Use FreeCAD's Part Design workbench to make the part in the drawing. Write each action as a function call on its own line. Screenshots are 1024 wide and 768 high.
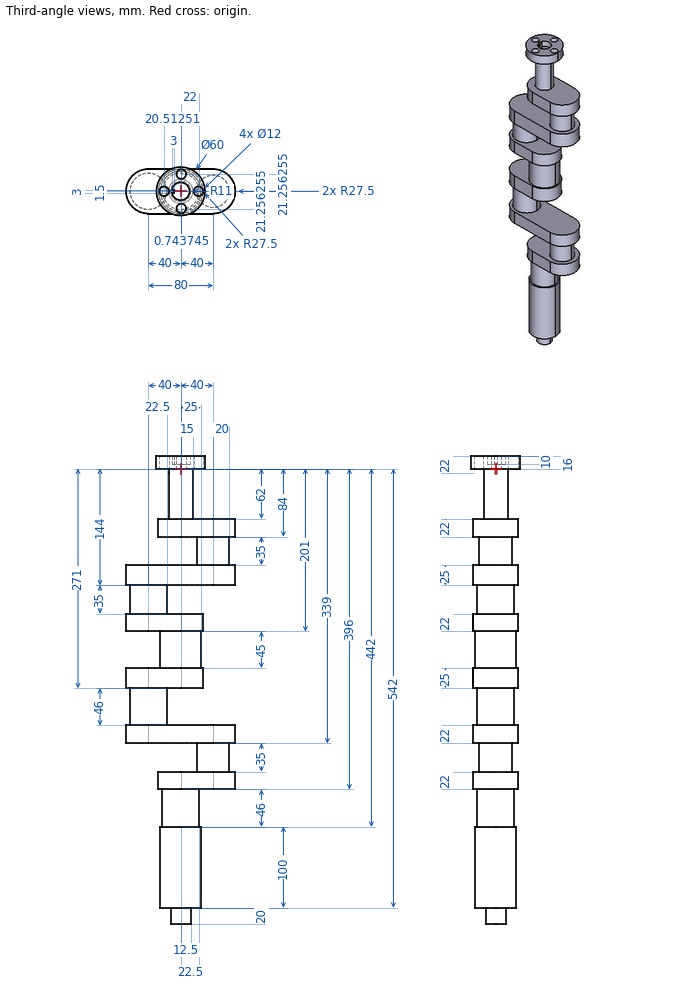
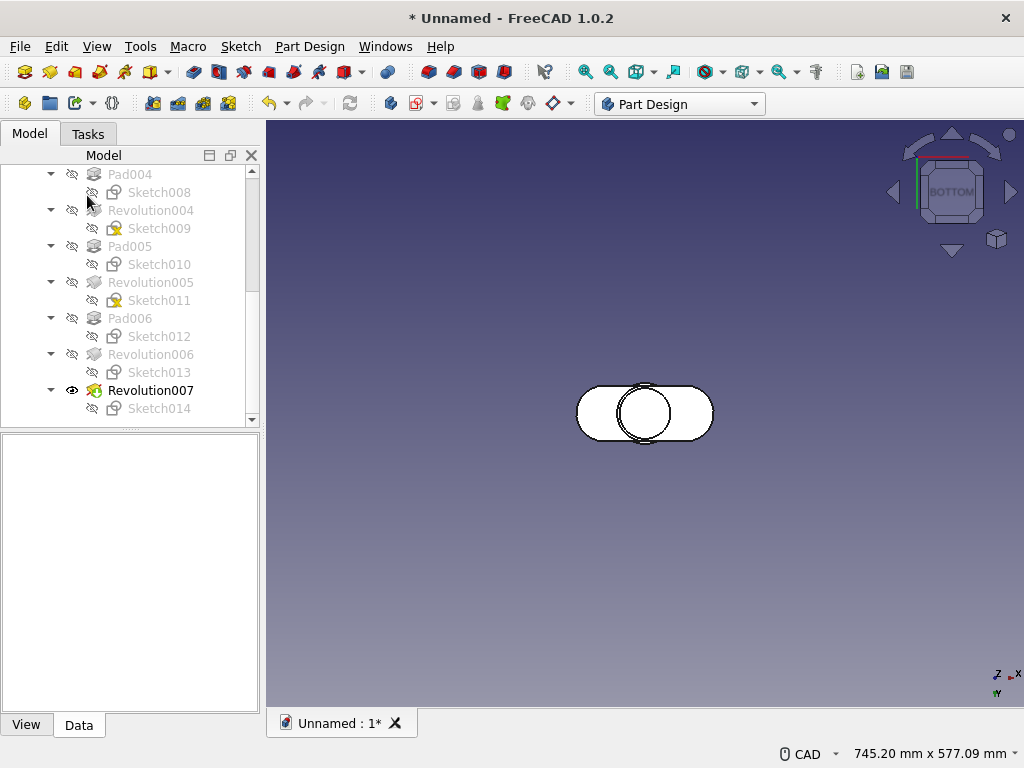
click(416, 104)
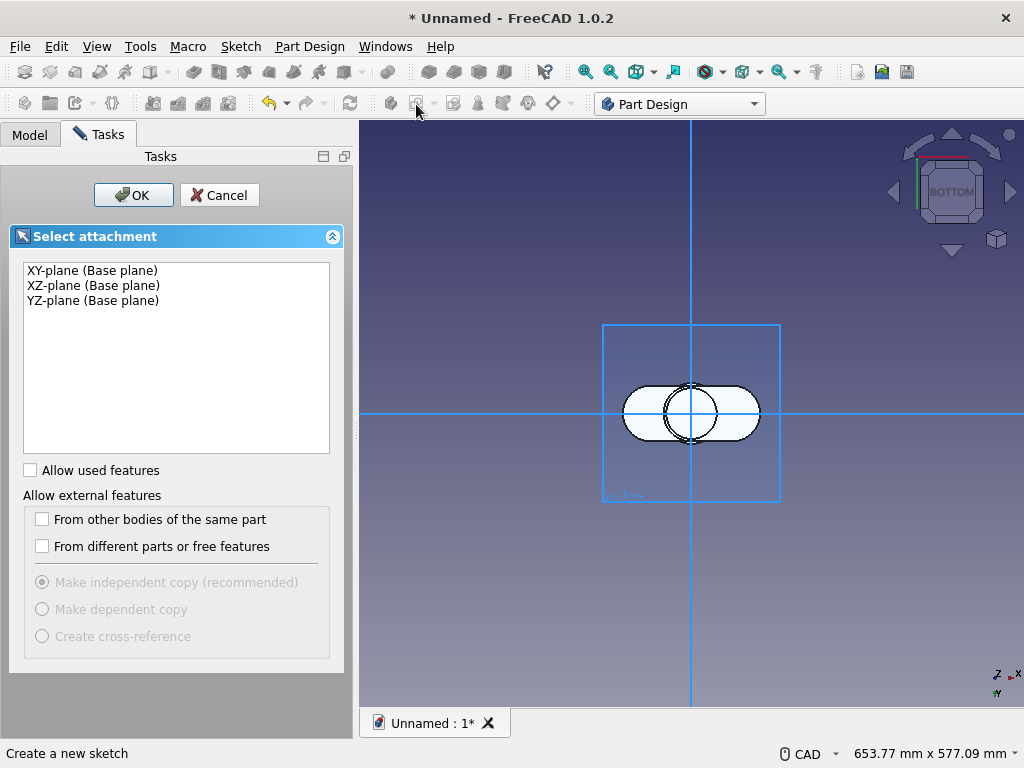
click(84, 286)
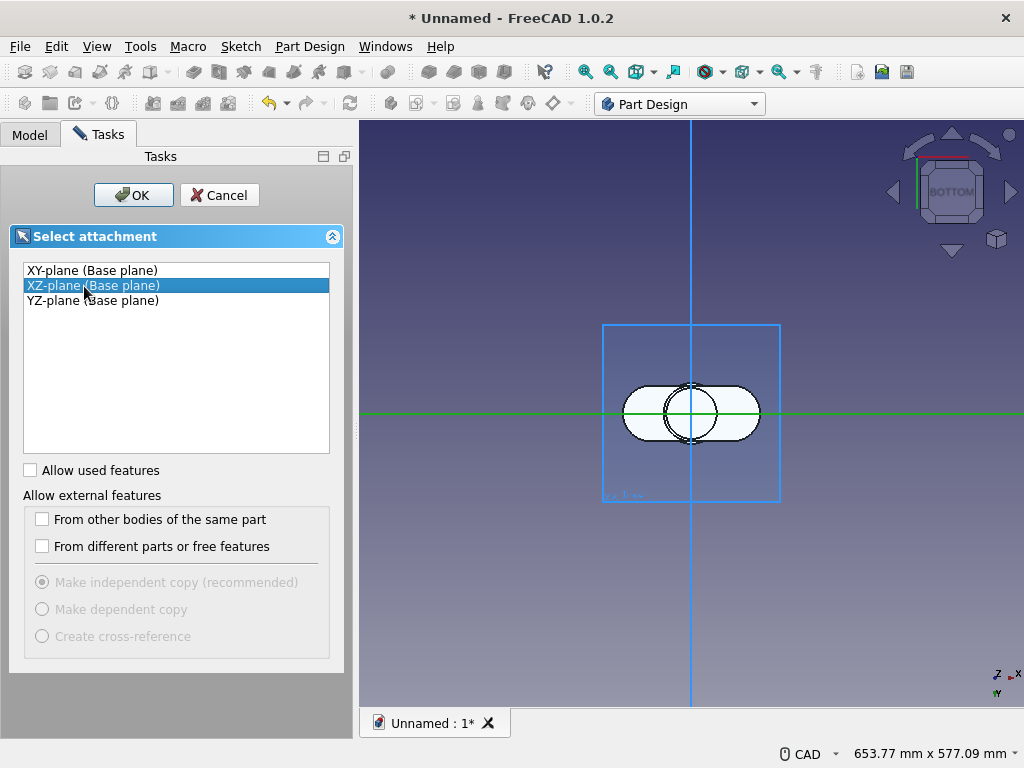
click(134, 195)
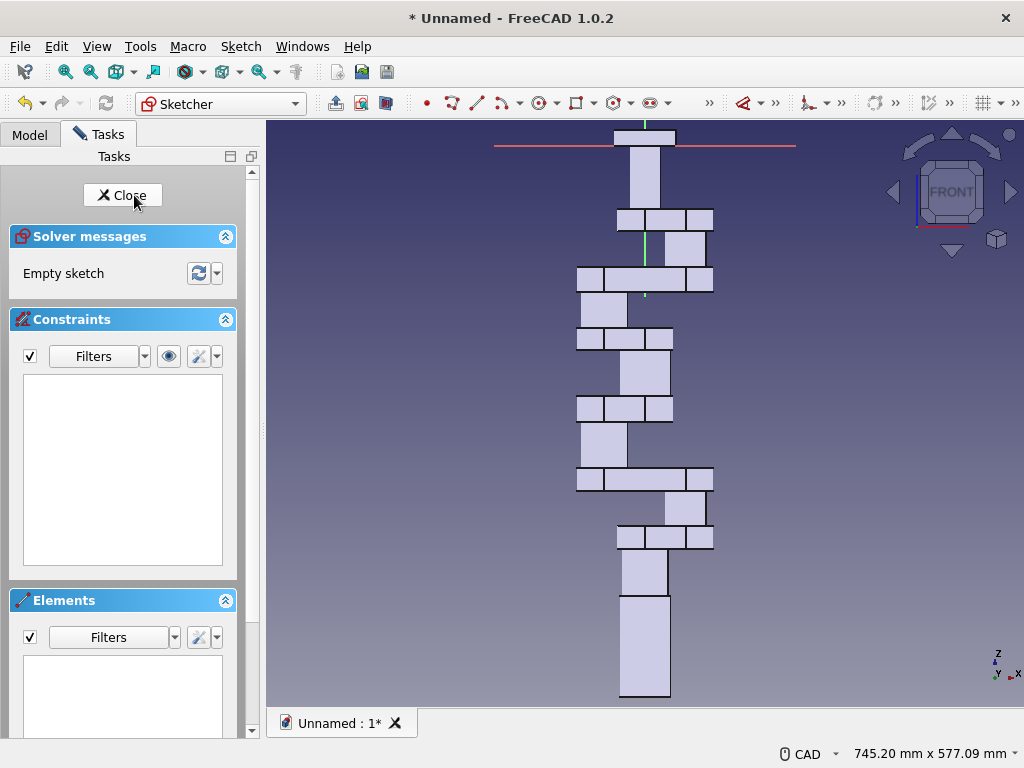
click(386, 104)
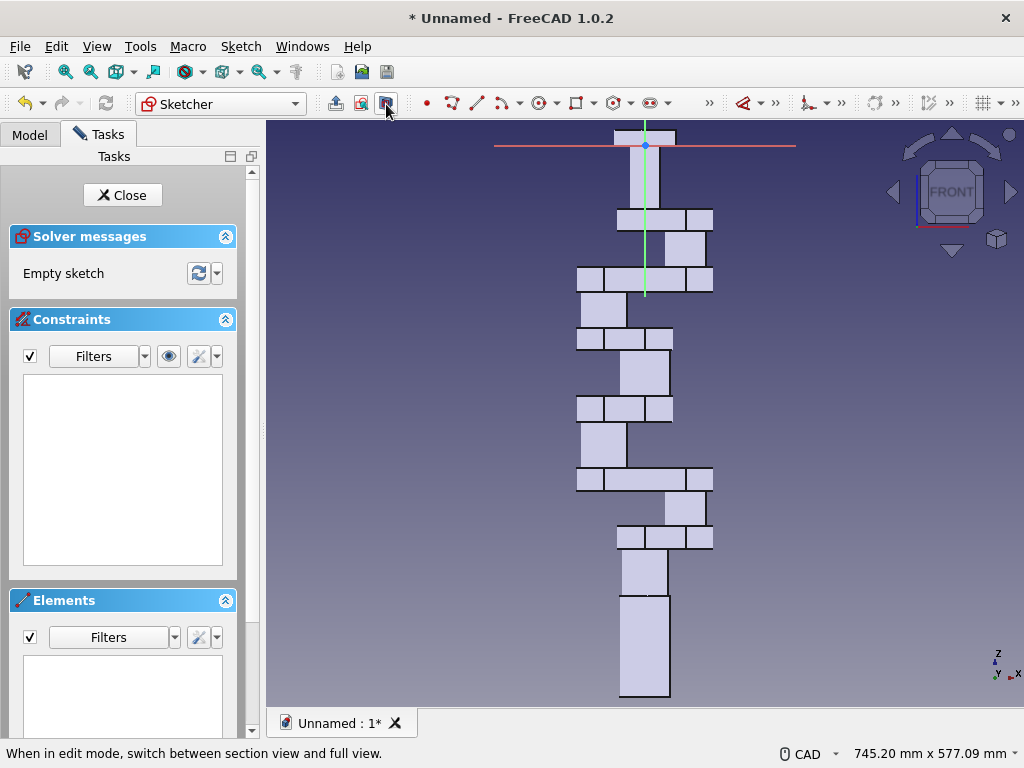
scroll(576, 414, down, 5)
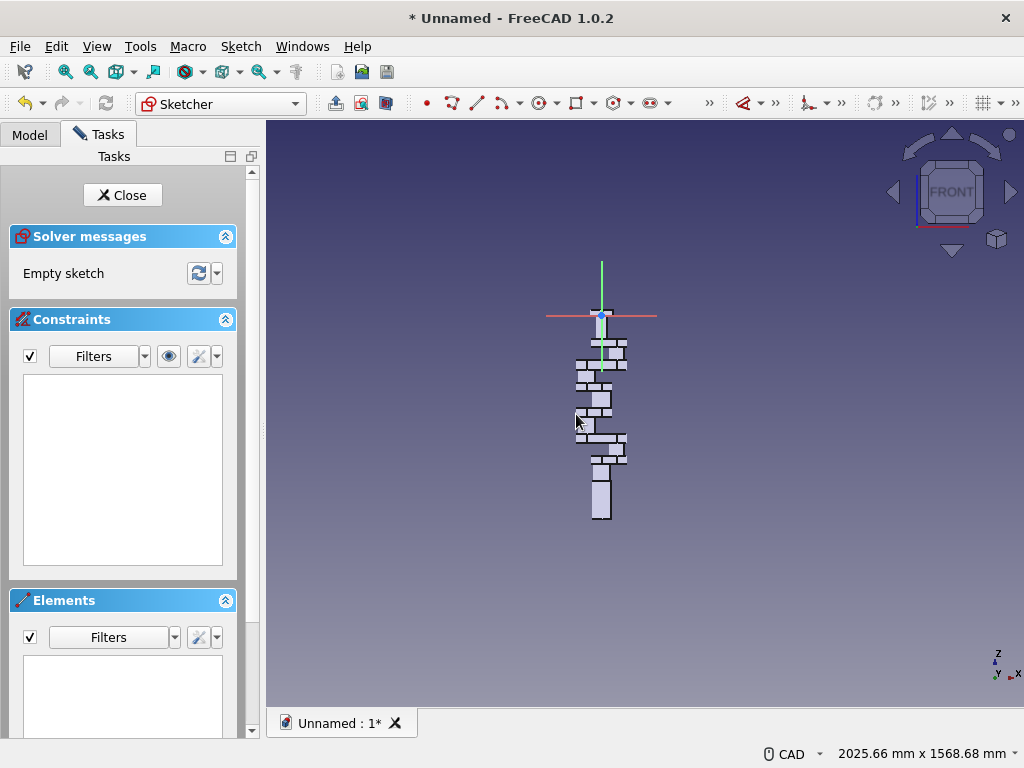
scroll(605, 528, up, 15)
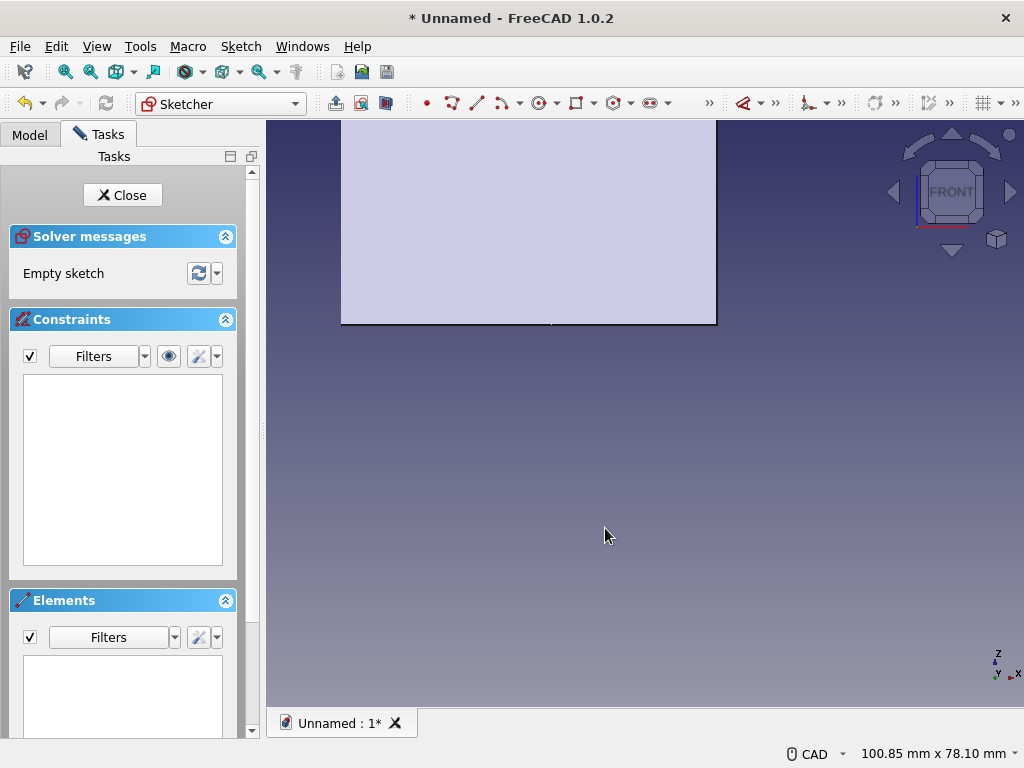
scroll(576, 392, up, 5)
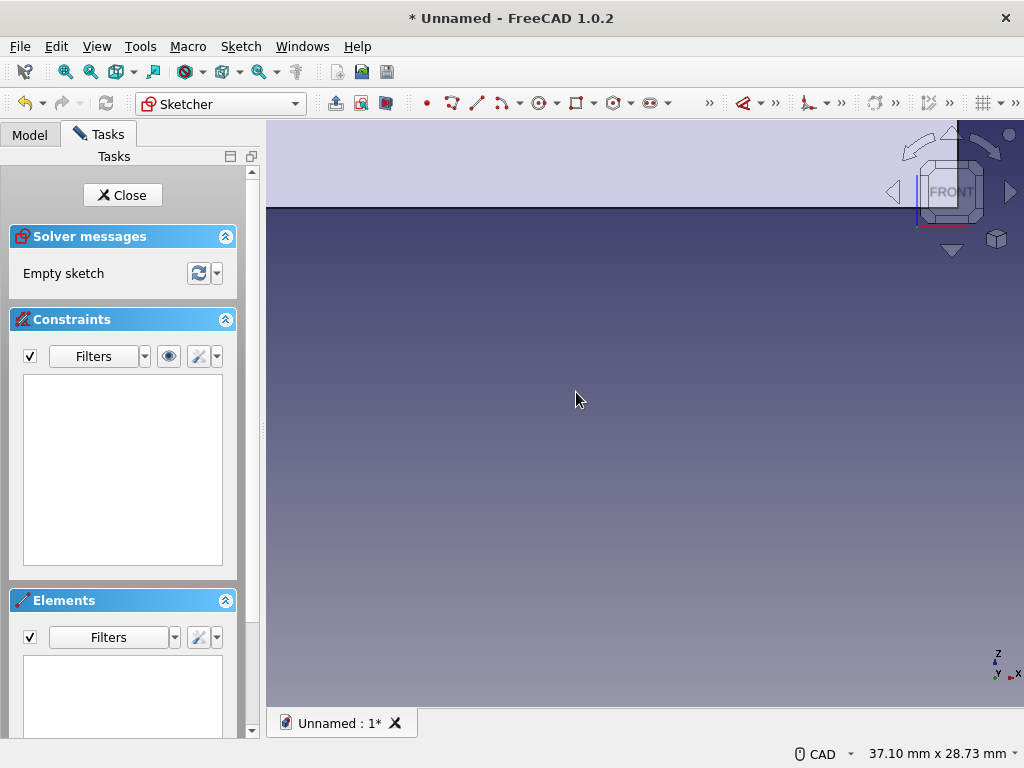
key(g)
key(r)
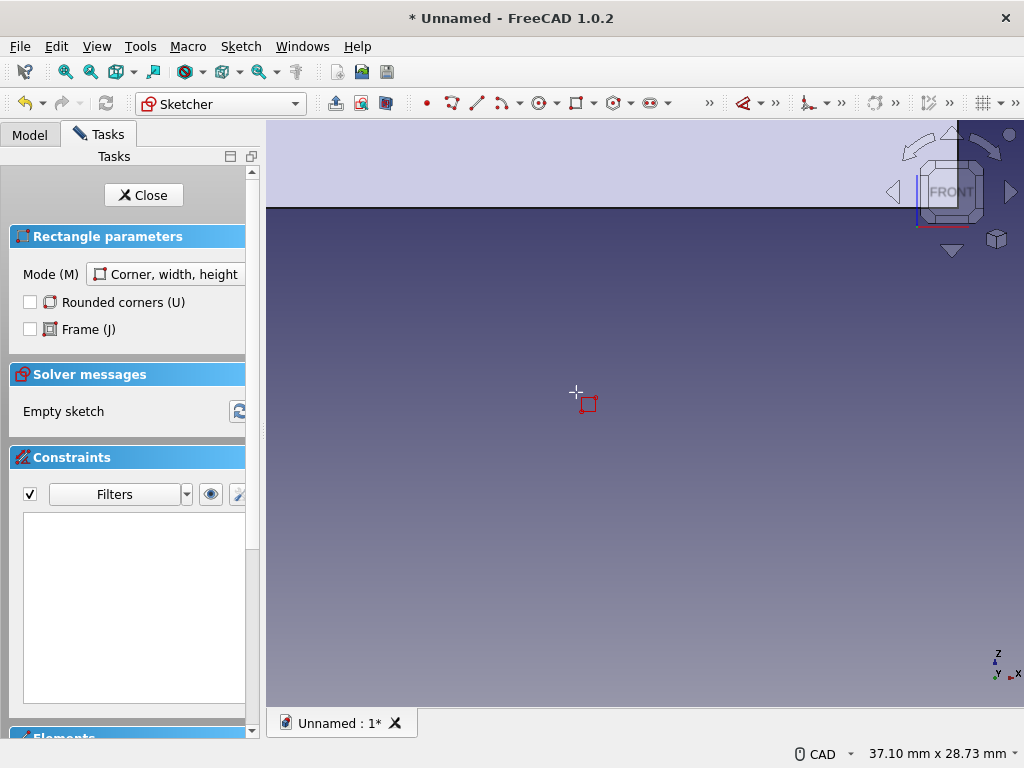
click(448, 208)
move(703, 617)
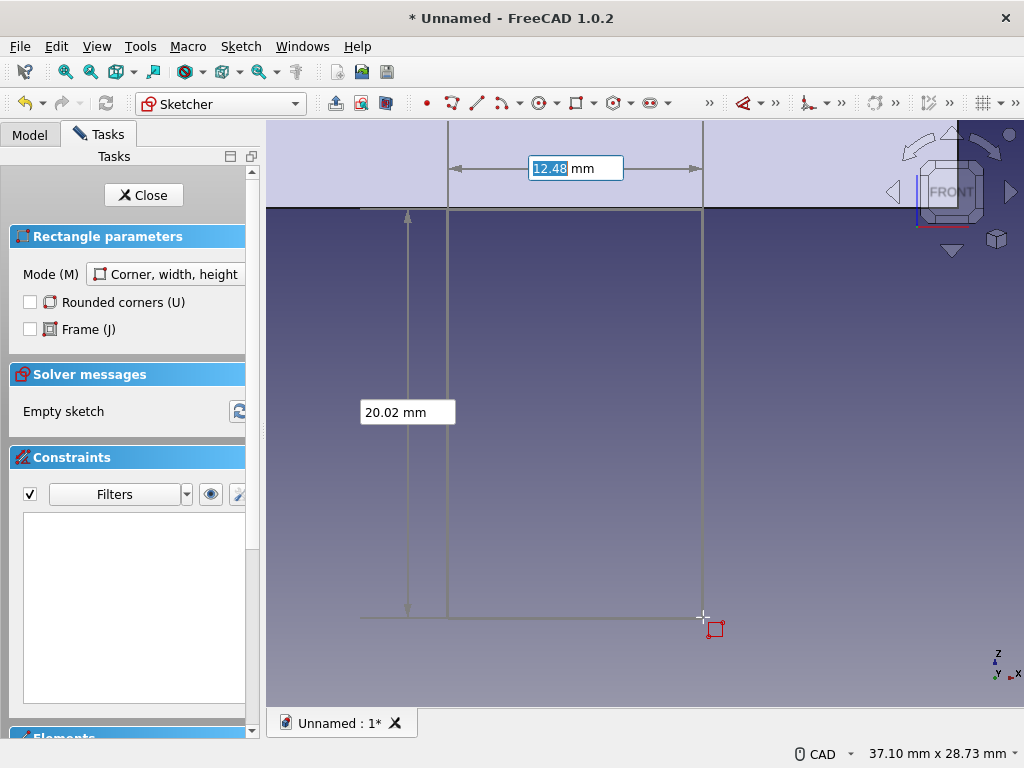
text(12.5)
key(Tab)
text(20)
key(Return)
key(Escape)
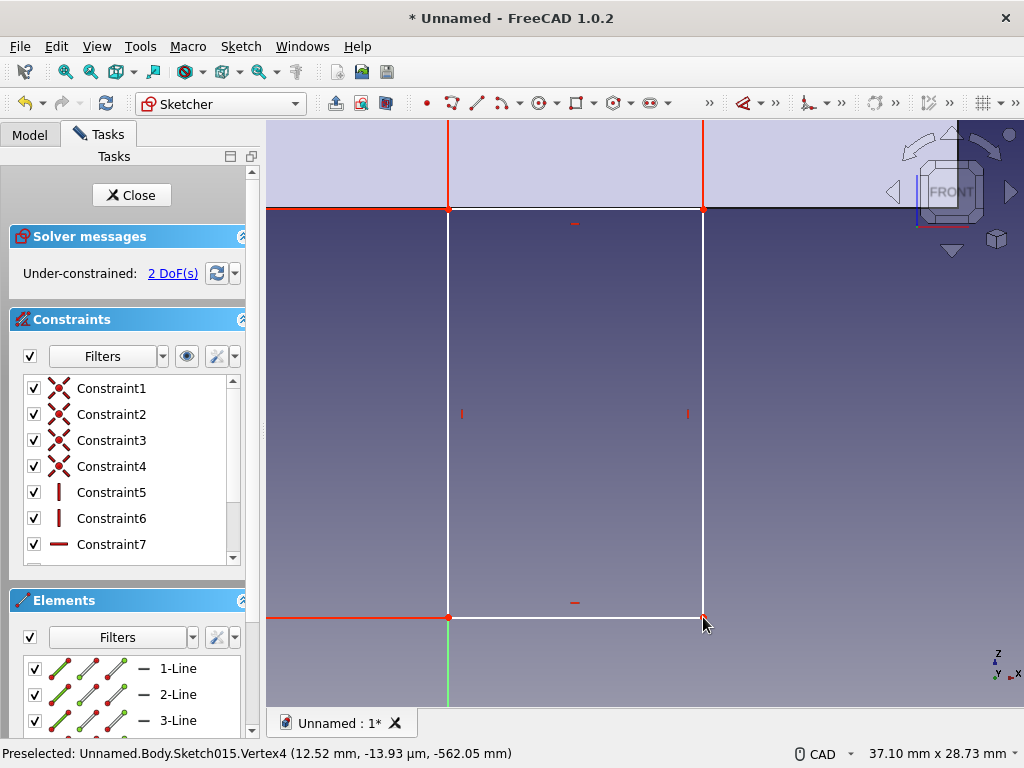
click(448, 209)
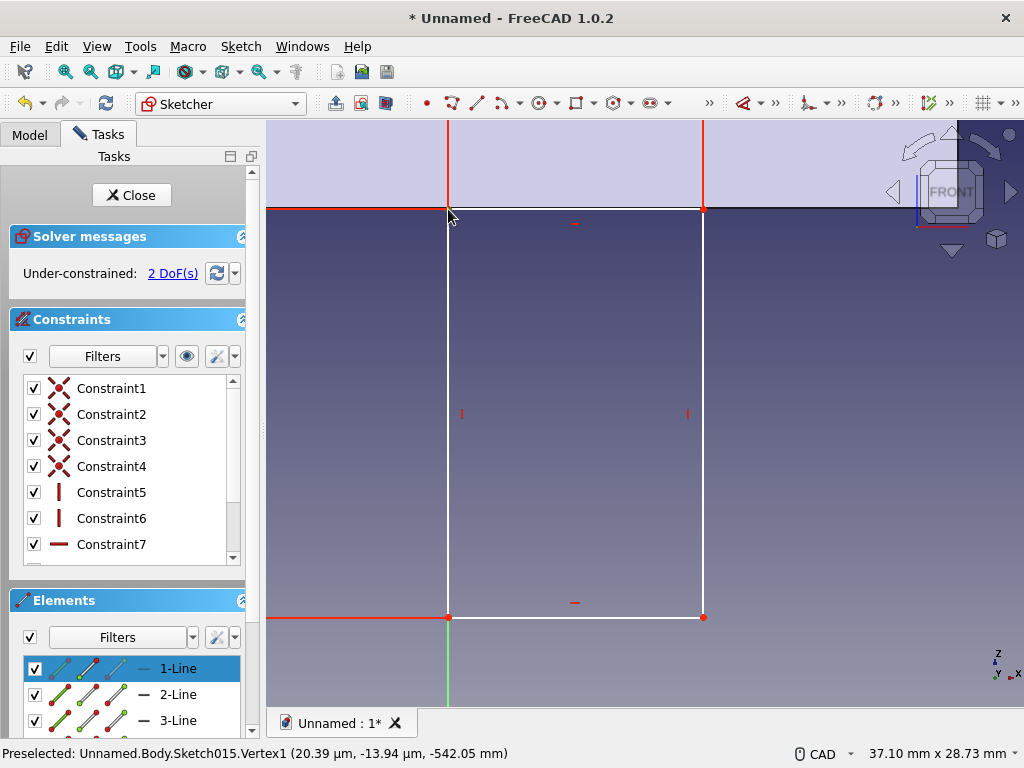
click(448, 641)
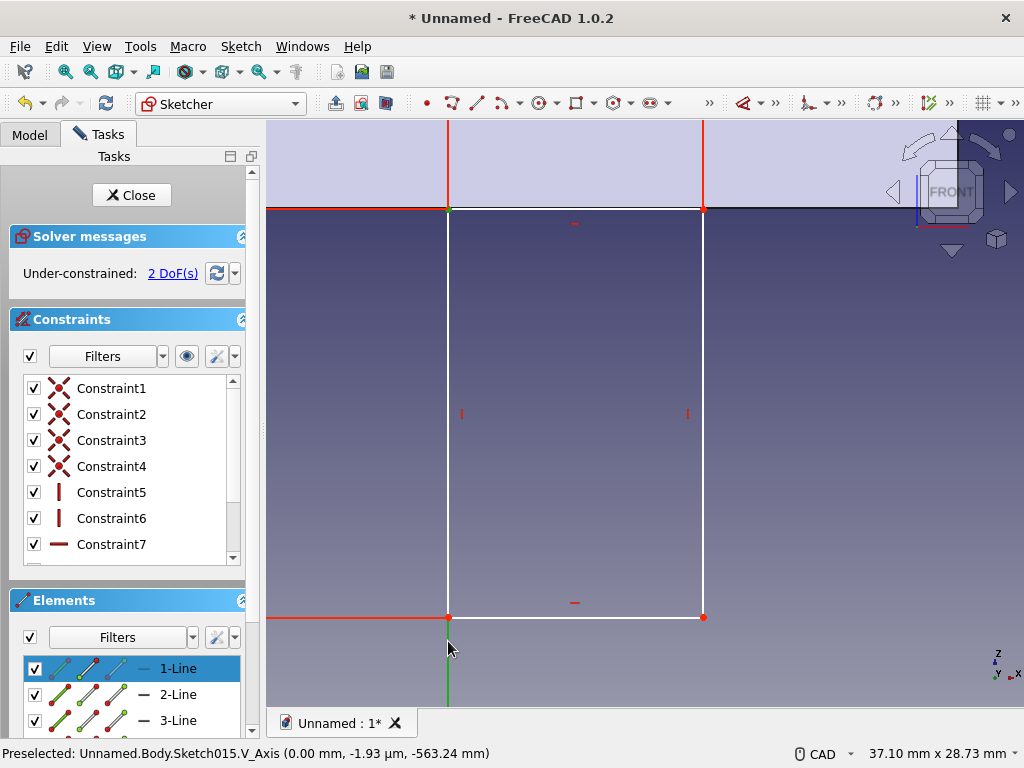
key(c)